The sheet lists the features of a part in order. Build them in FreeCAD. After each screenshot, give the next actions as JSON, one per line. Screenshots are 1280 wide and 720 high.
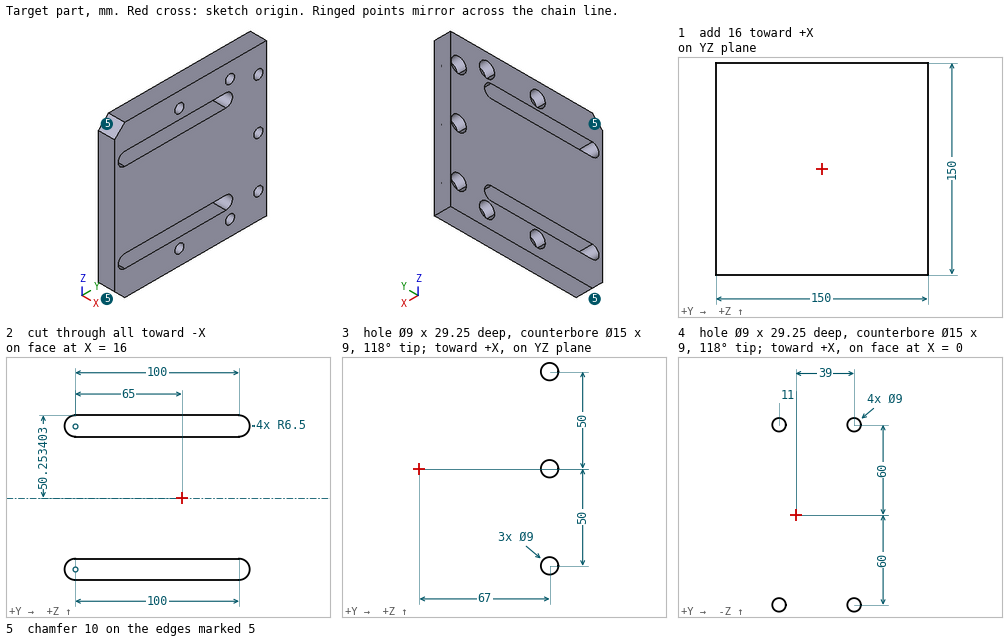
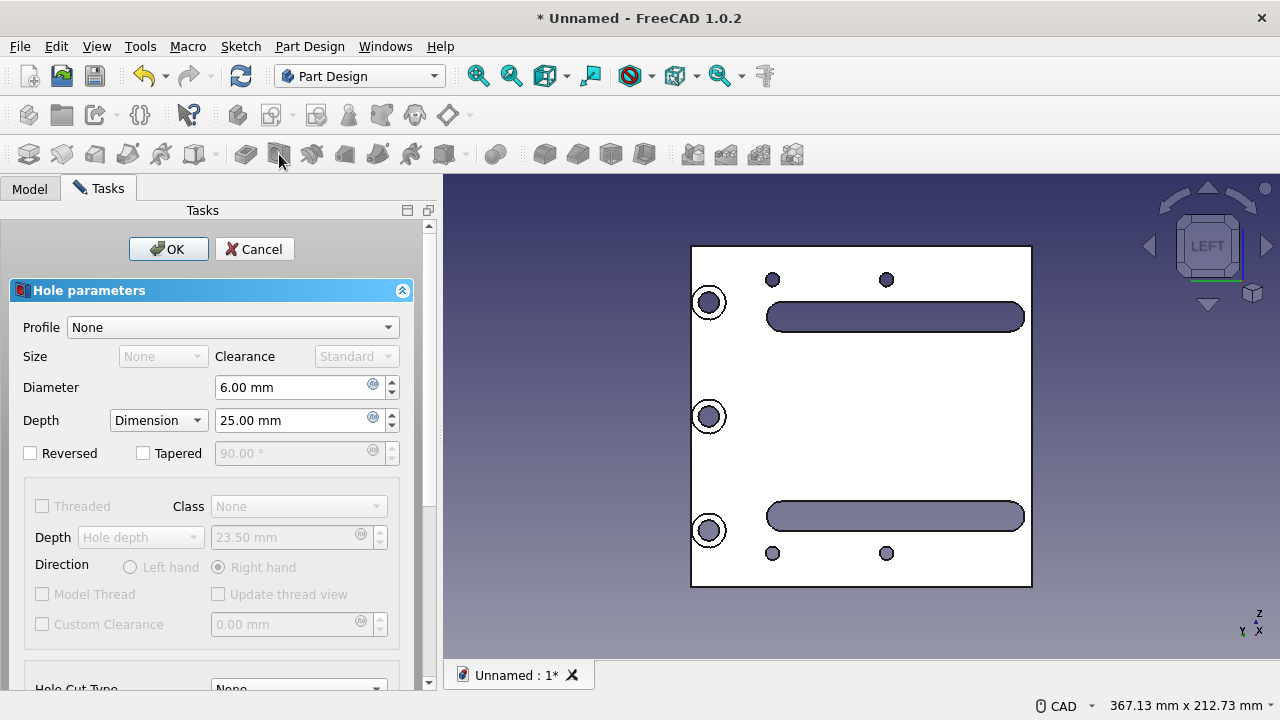
{"action": "triple_click", "coordinate": [300, 388]}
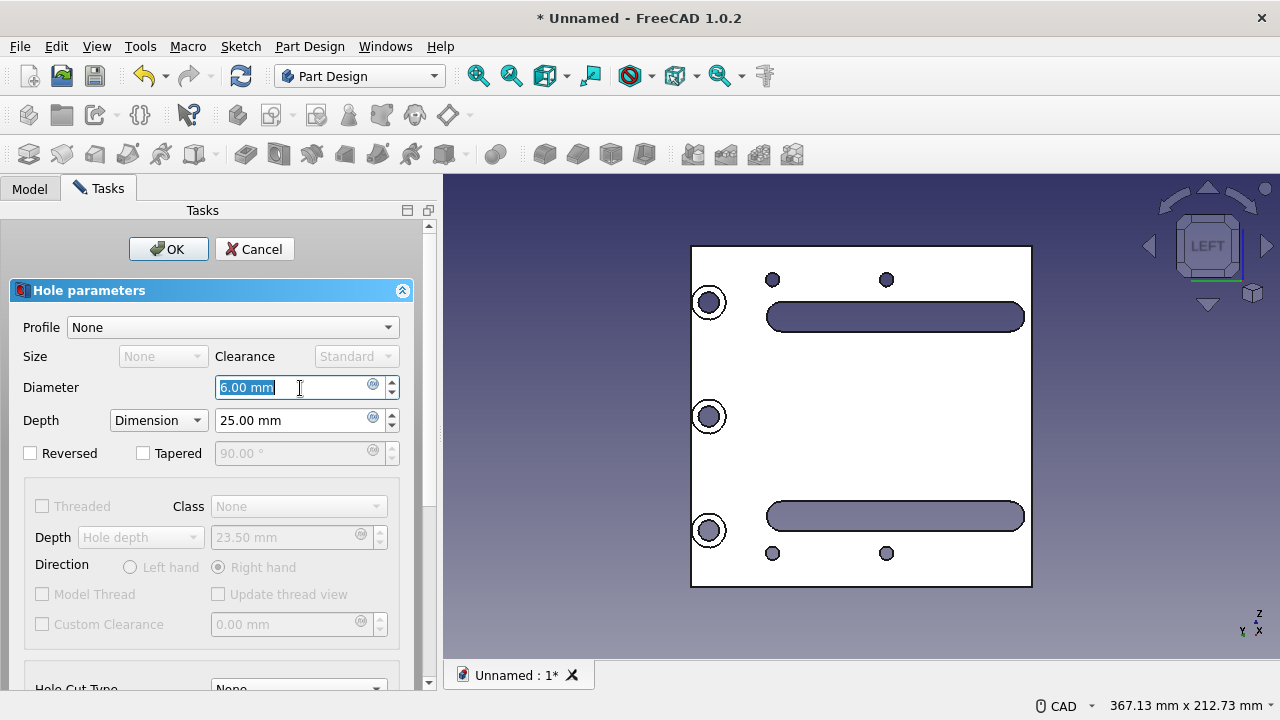
{"action": "type", "text": "9"}
{"action": "key", "text": "Tab"}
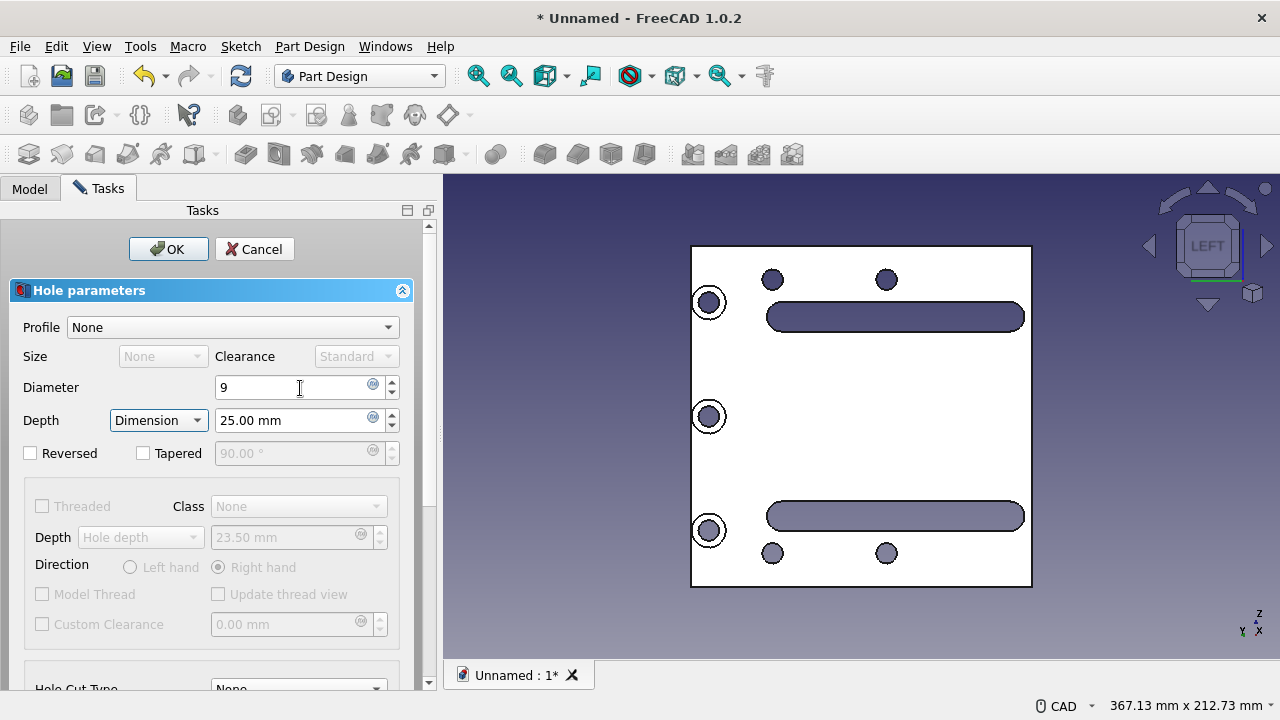
{"action": "triple_click", "coordinate": [300, 420]}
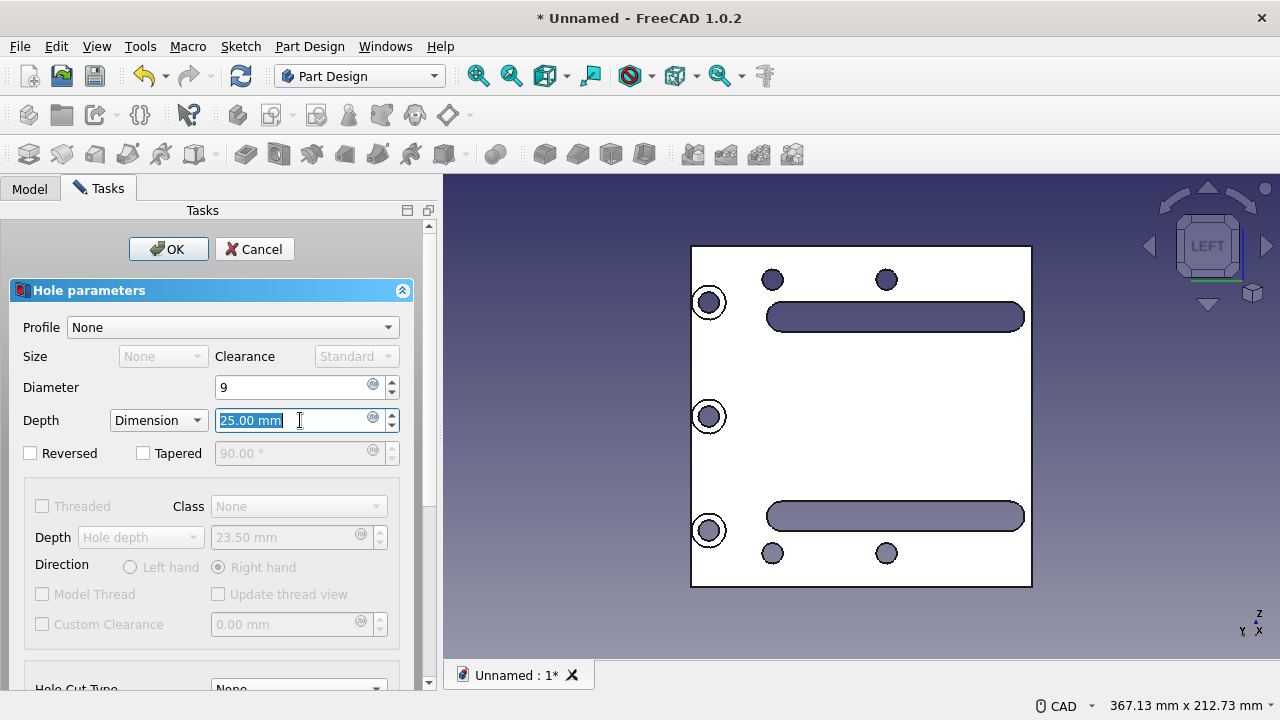
{"action": "type", "text": "29.25"}
{"action": "key", "text": "Tab"}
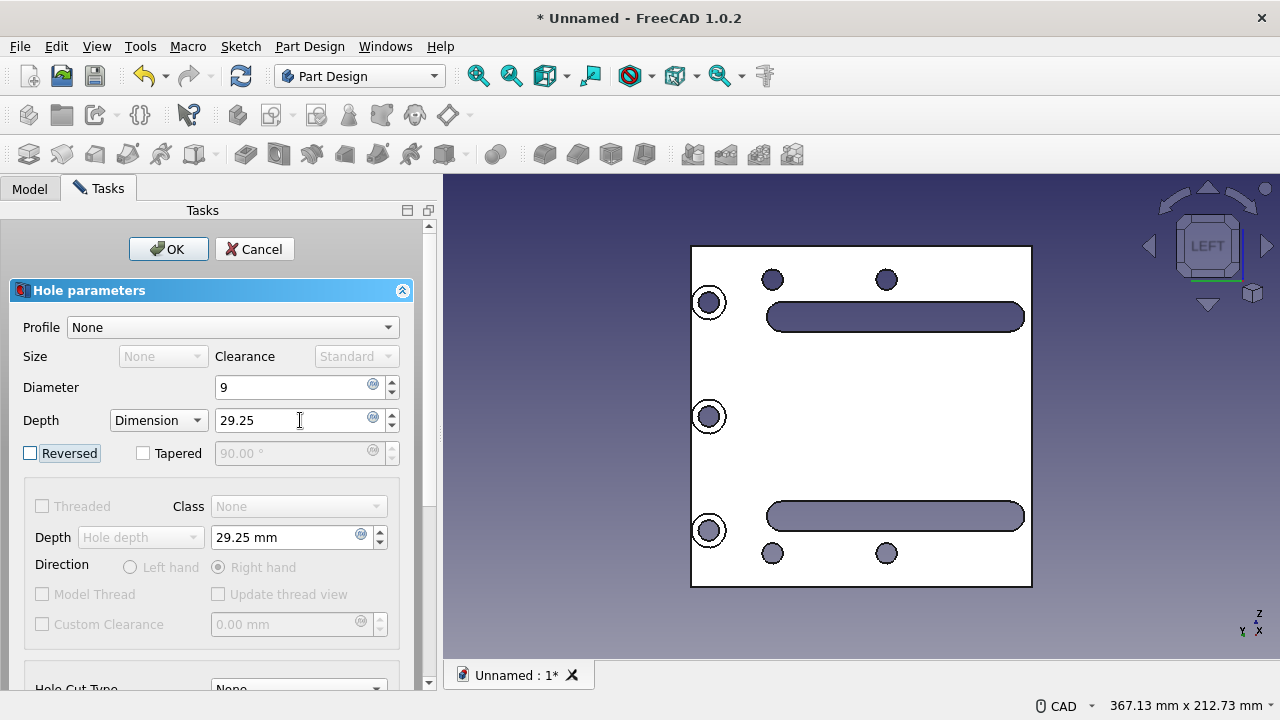
{"action": "scroll", "coordinate": [429, 455], "scroll_direction": "down", "scroll_amount": 2}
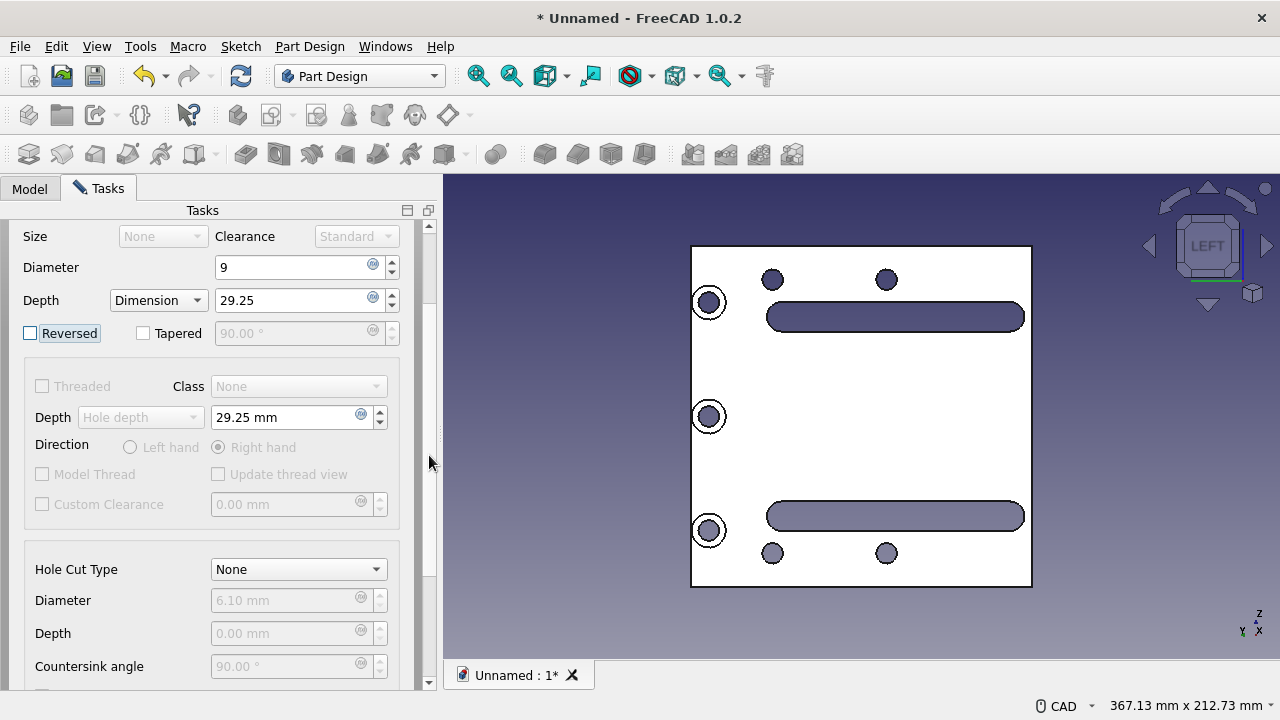
{"action": "left_click", "coordinate": [300, 570]}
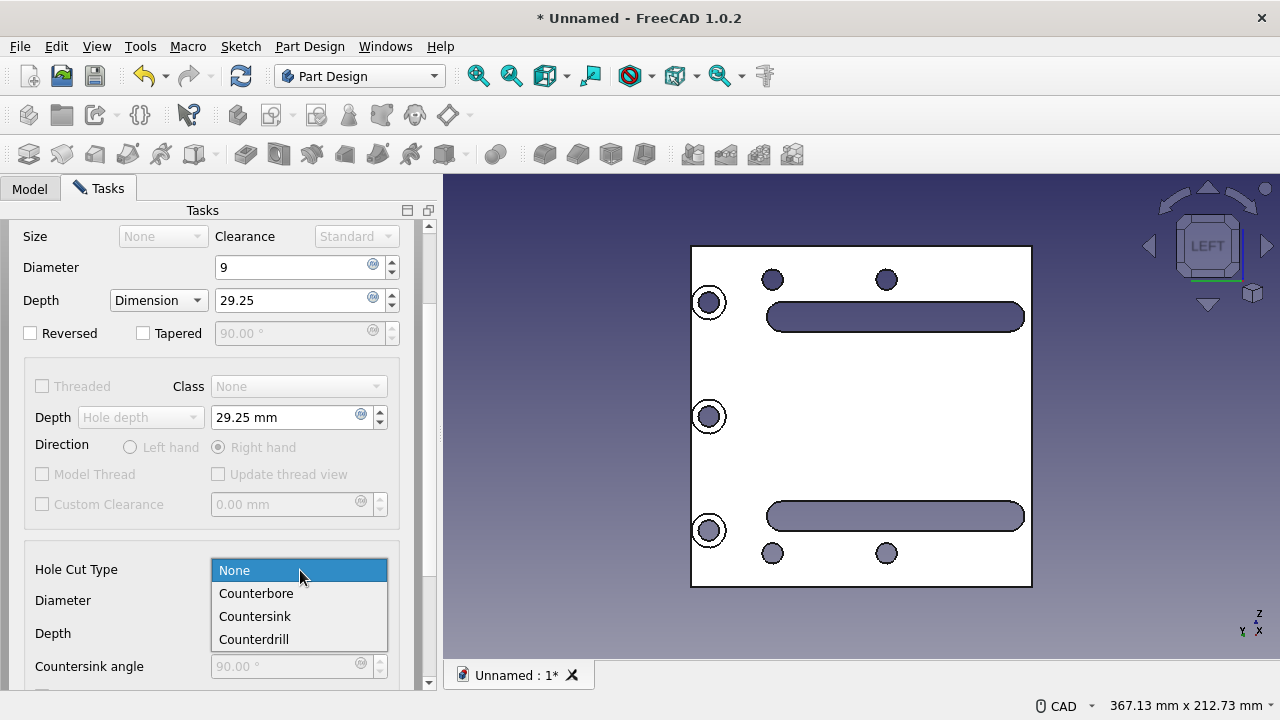
{"action": "left_click", "coordinate": [298, 594]}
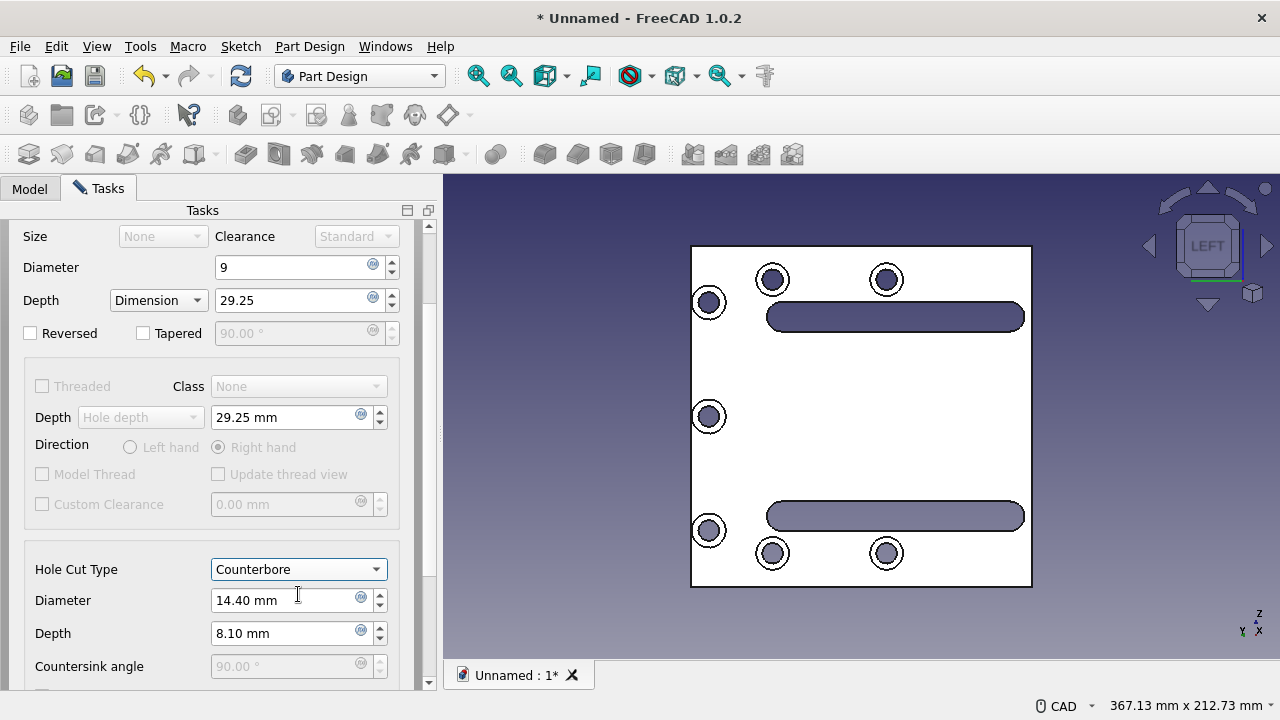
{"action": "triple_click", "coordinate": [292, 600]}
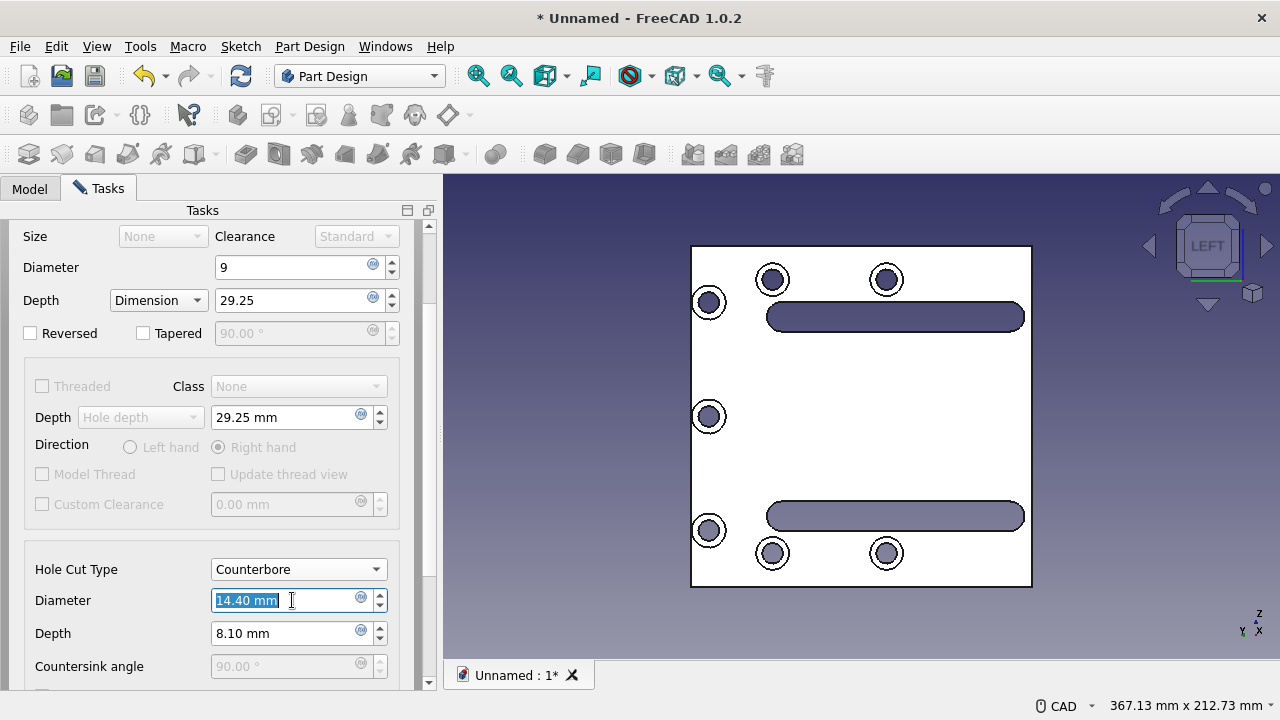
{"action": "type", "text": "15"}
{"action": "key", "text": "Tab"}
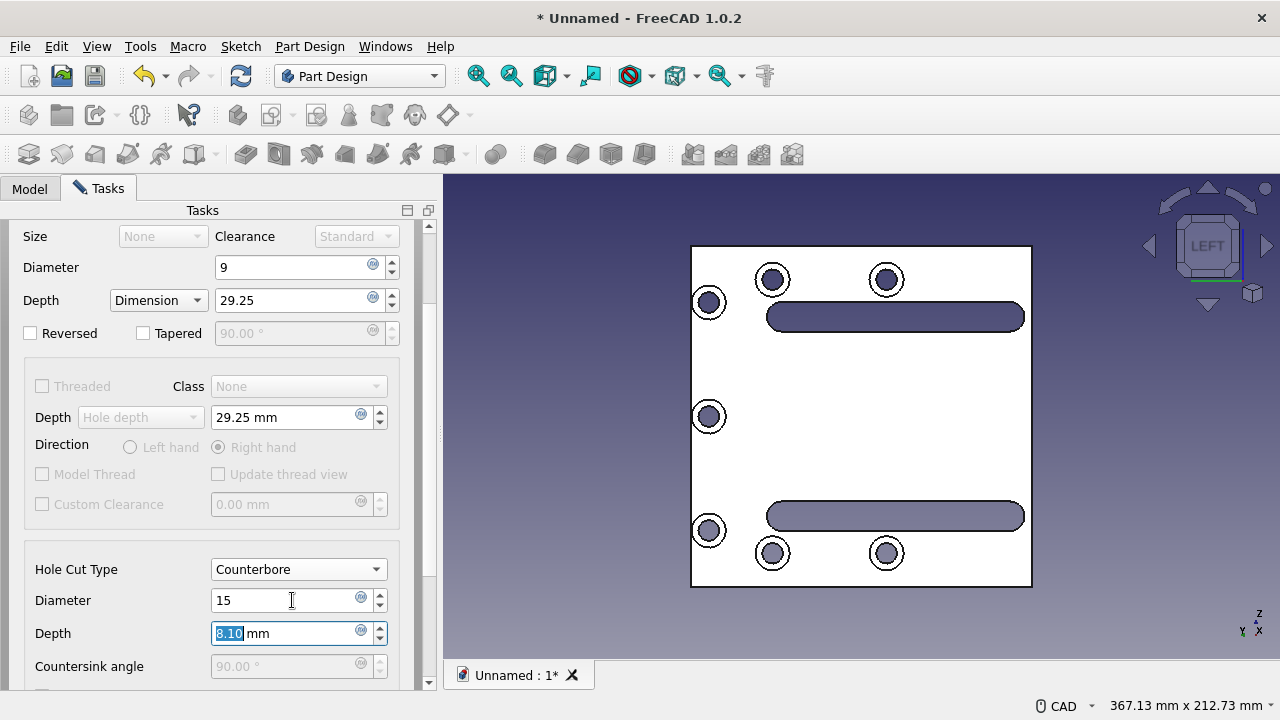
{"action": "type", "text": "9"}
{"action": "key", "text": "Tab"}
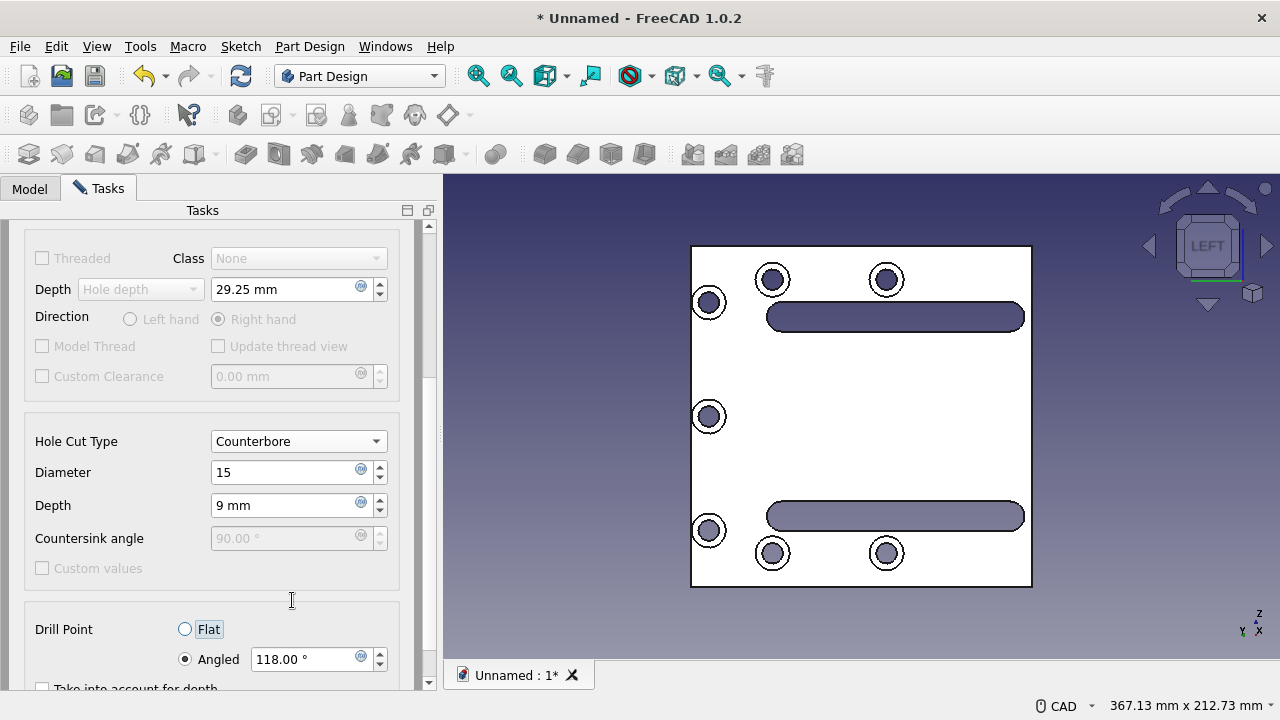
{"action": "scroll", "coordinate": [429, 455], "scroll_direction": "up", "scroll_amount": 5}